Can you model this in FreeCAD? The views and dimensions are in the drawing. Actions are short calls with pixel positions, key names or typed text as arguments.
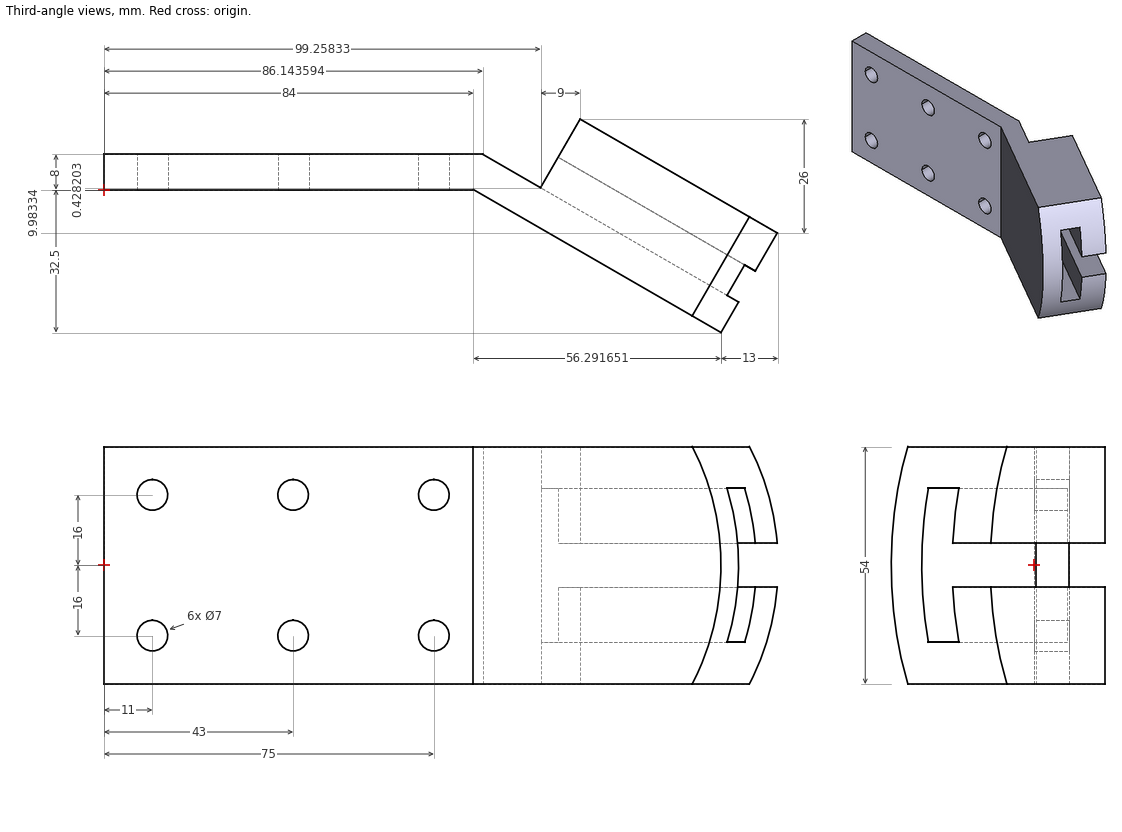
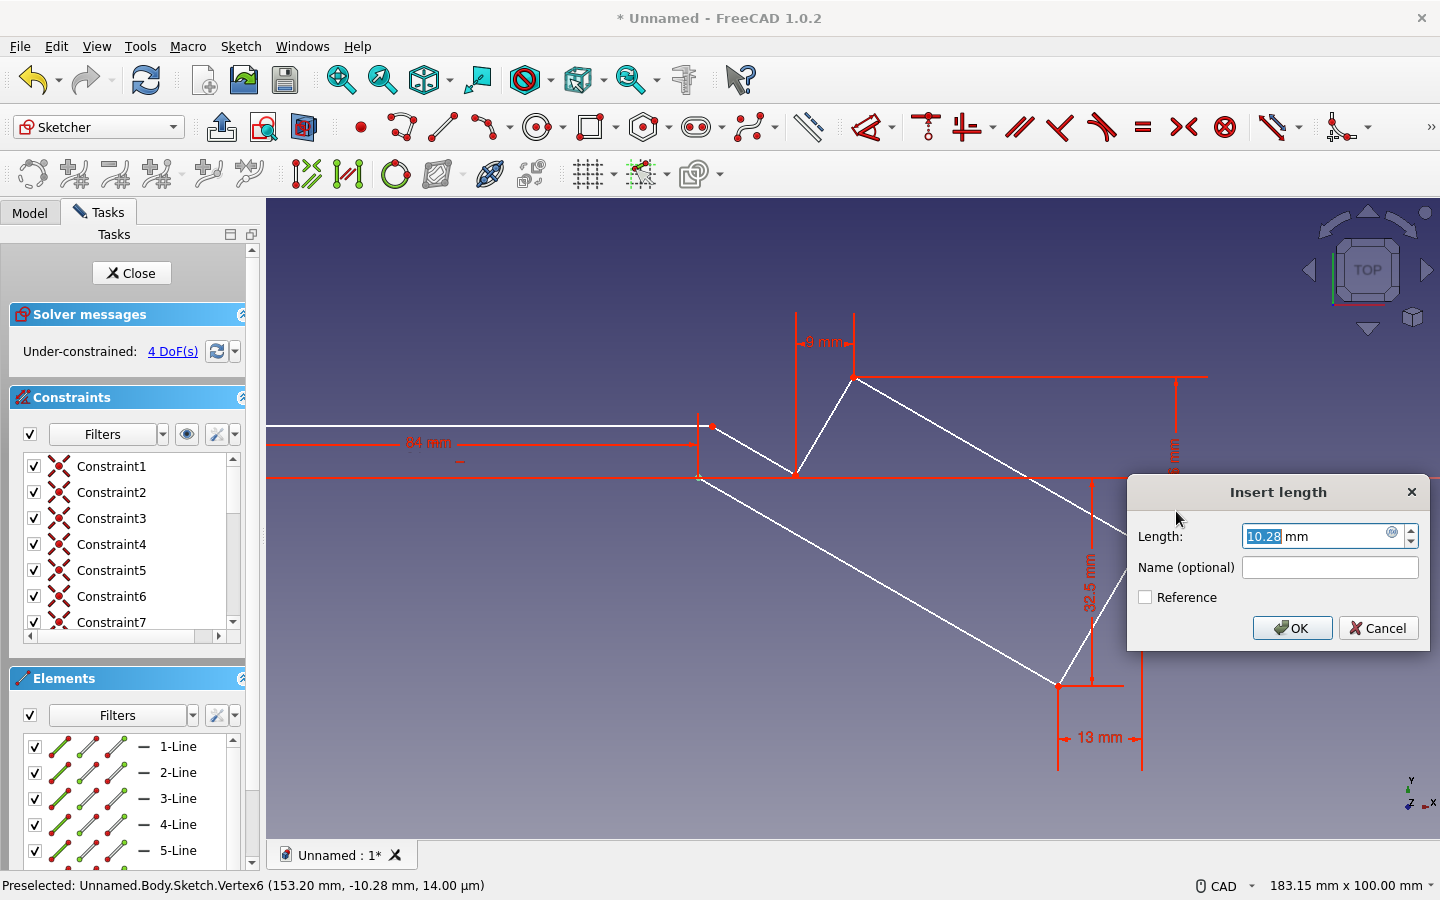
text(9.98334)
key(Return)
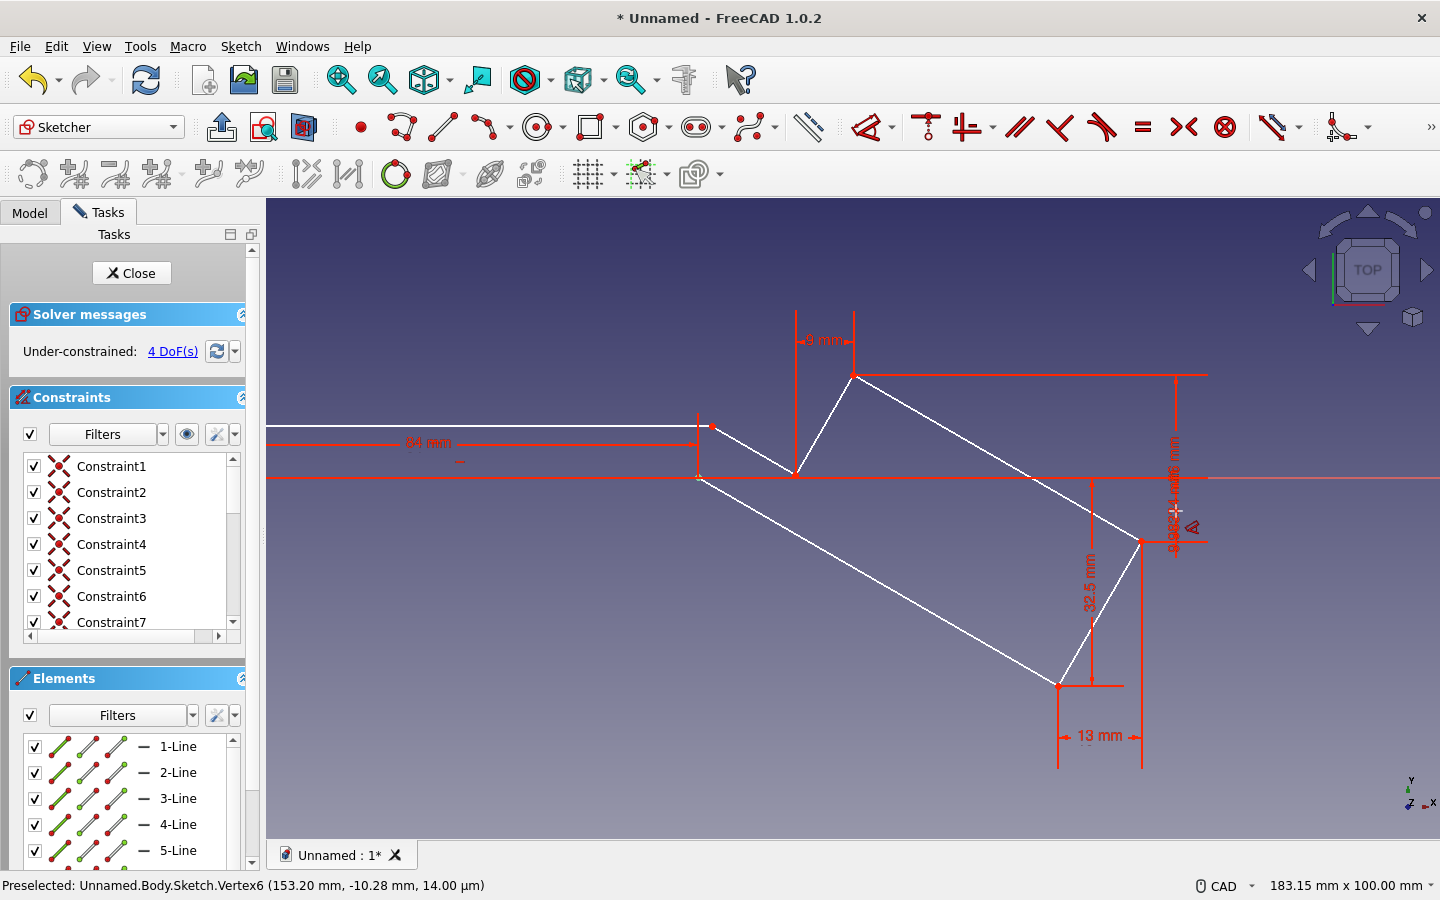
click(546, 426)
click(503, 392)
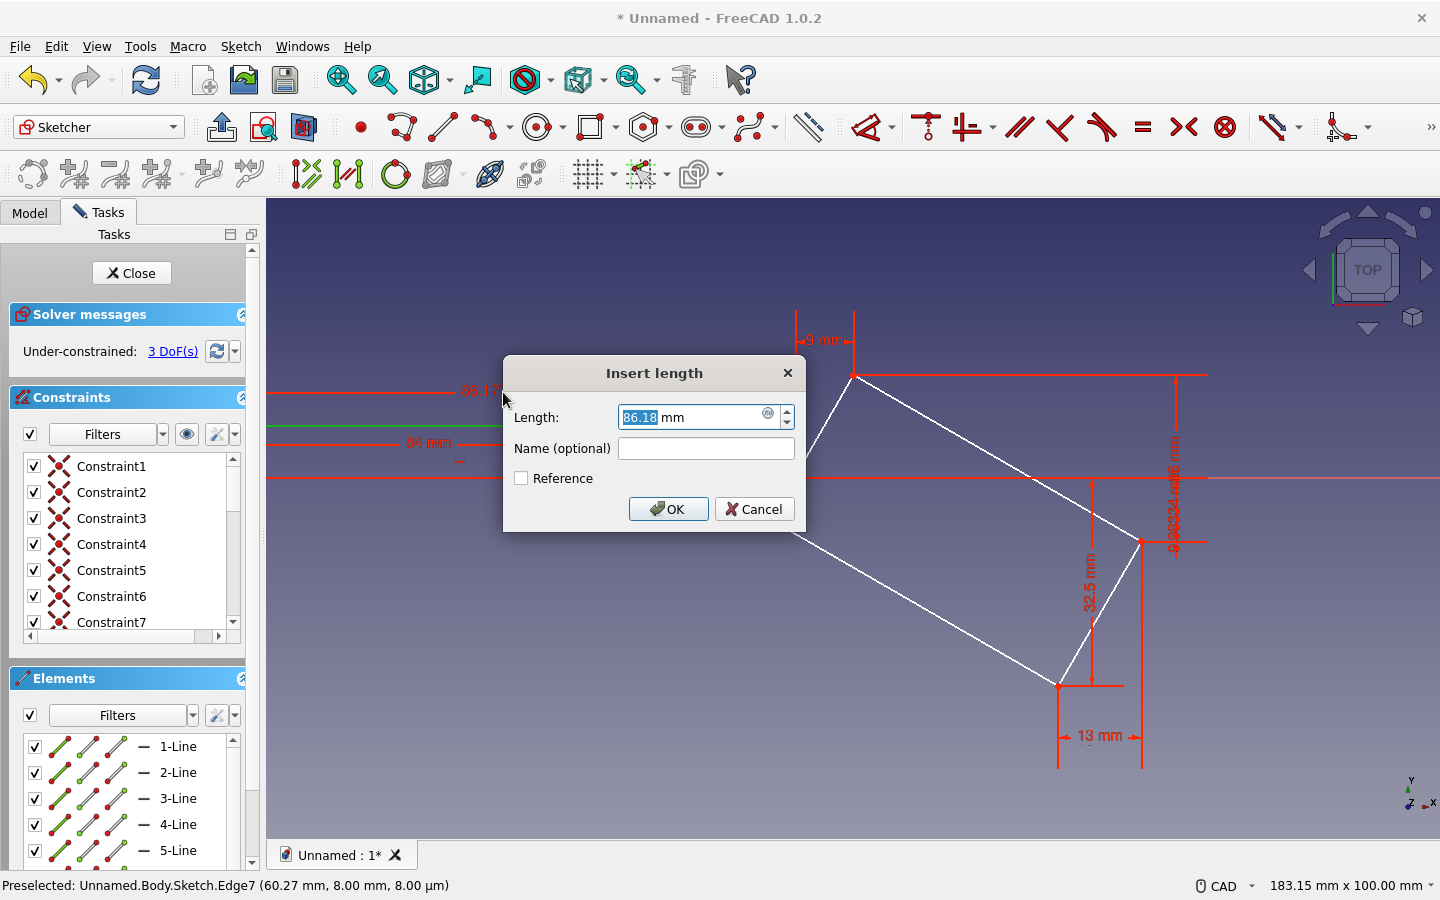
text(86.143594)
key(Return)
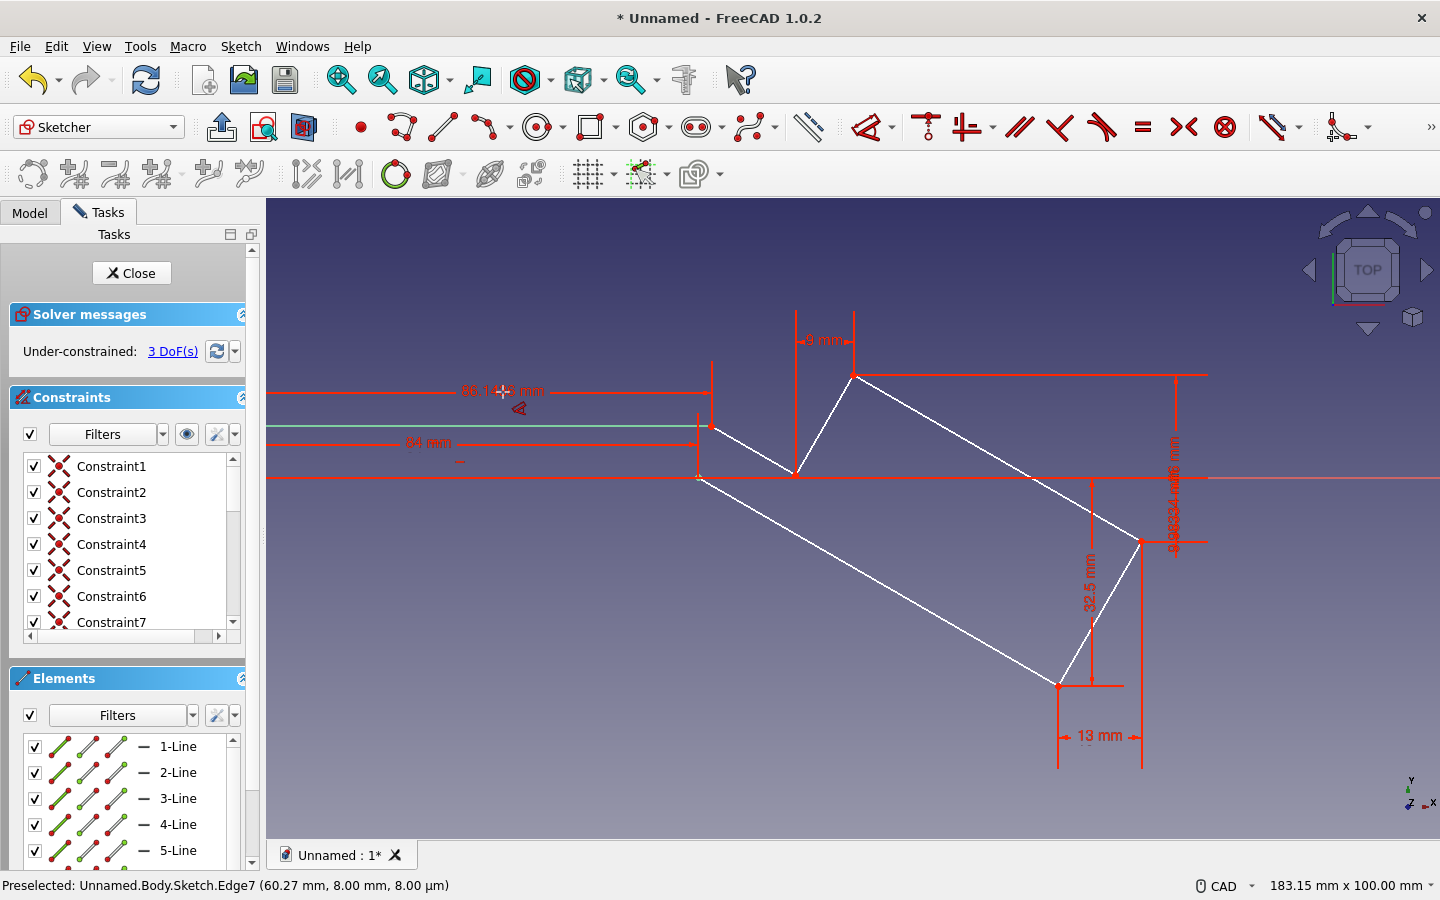
click(796, 475)
click(545, 441)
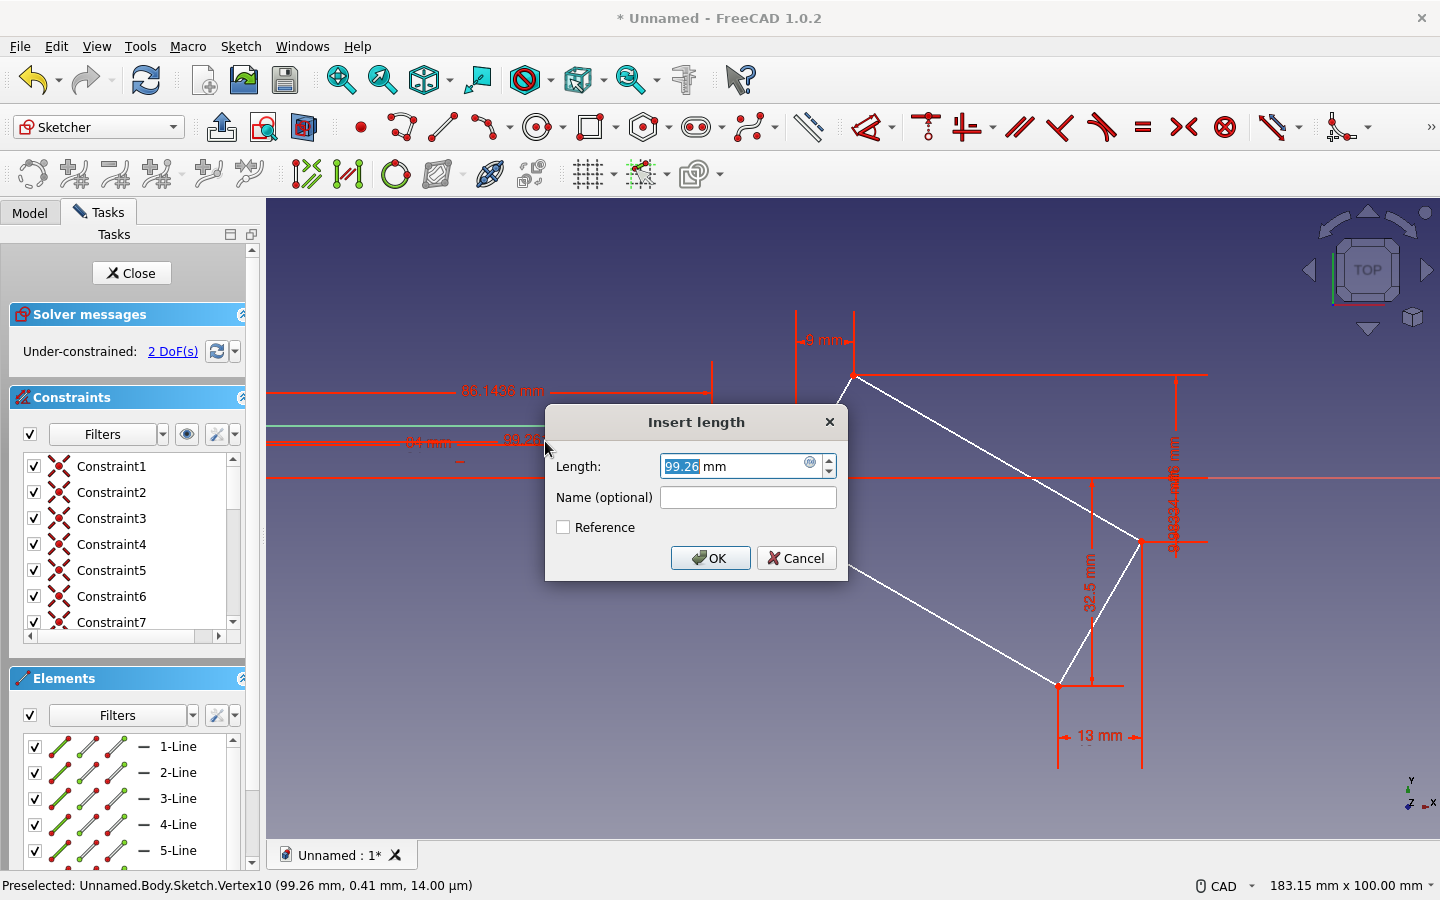
text(99.25833)
key(Return)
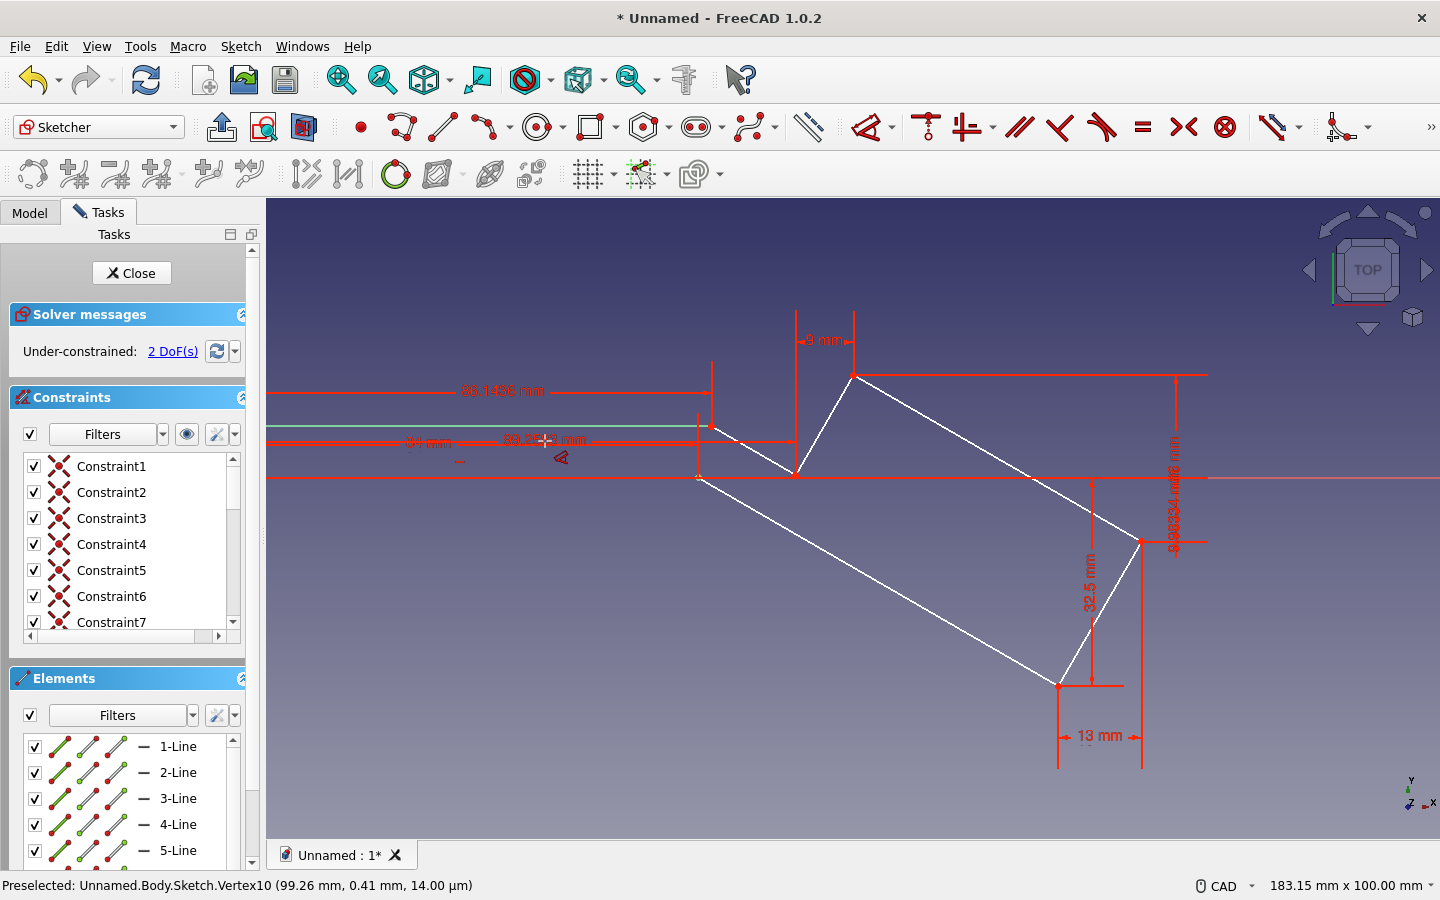
scroll(796, 475, up, 14)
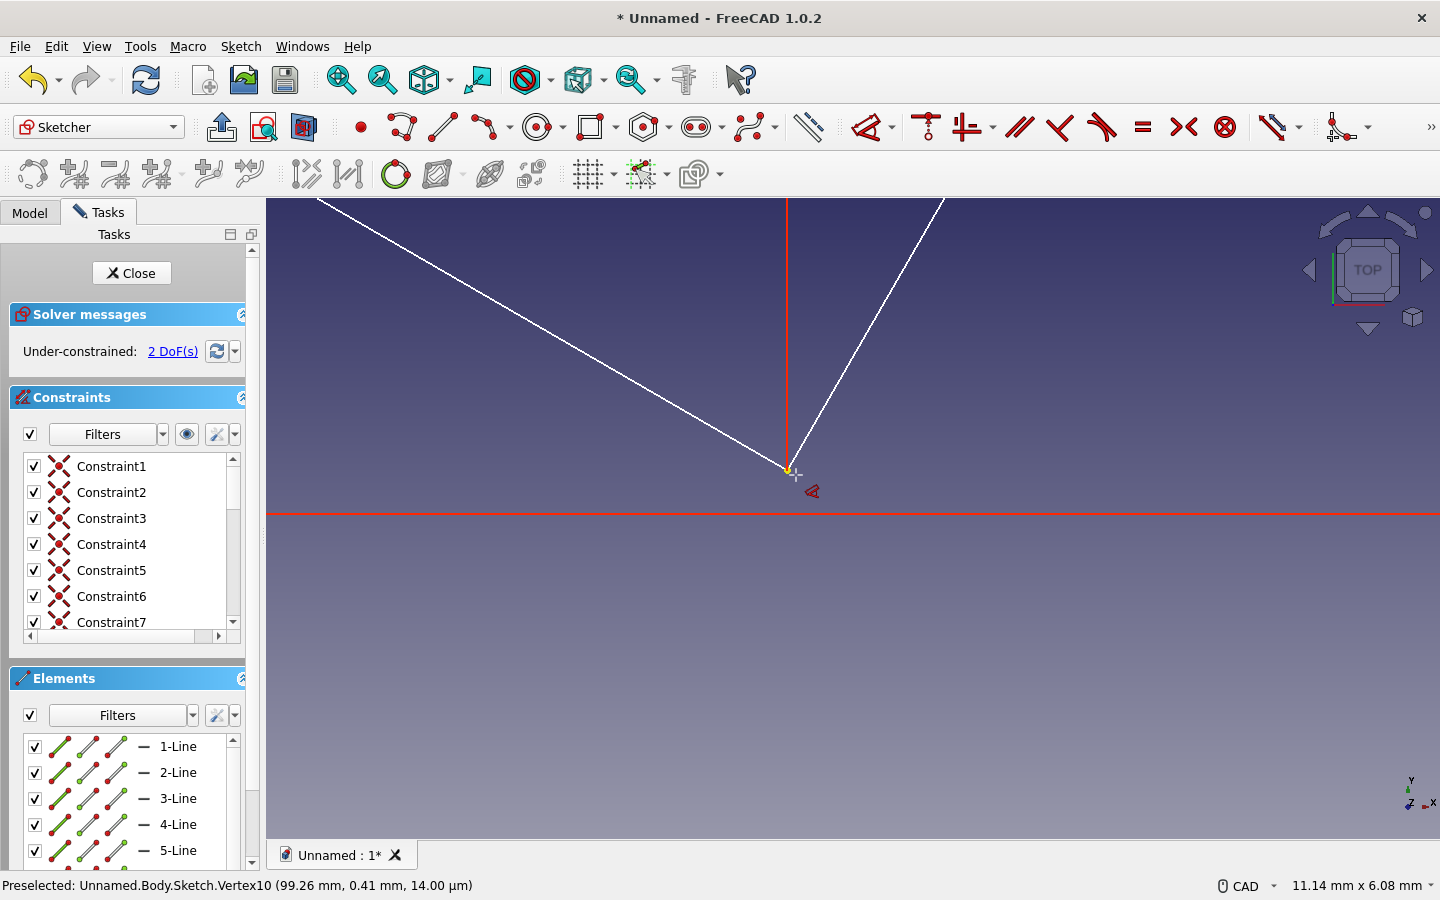
click(787, 471)
click(821, 492)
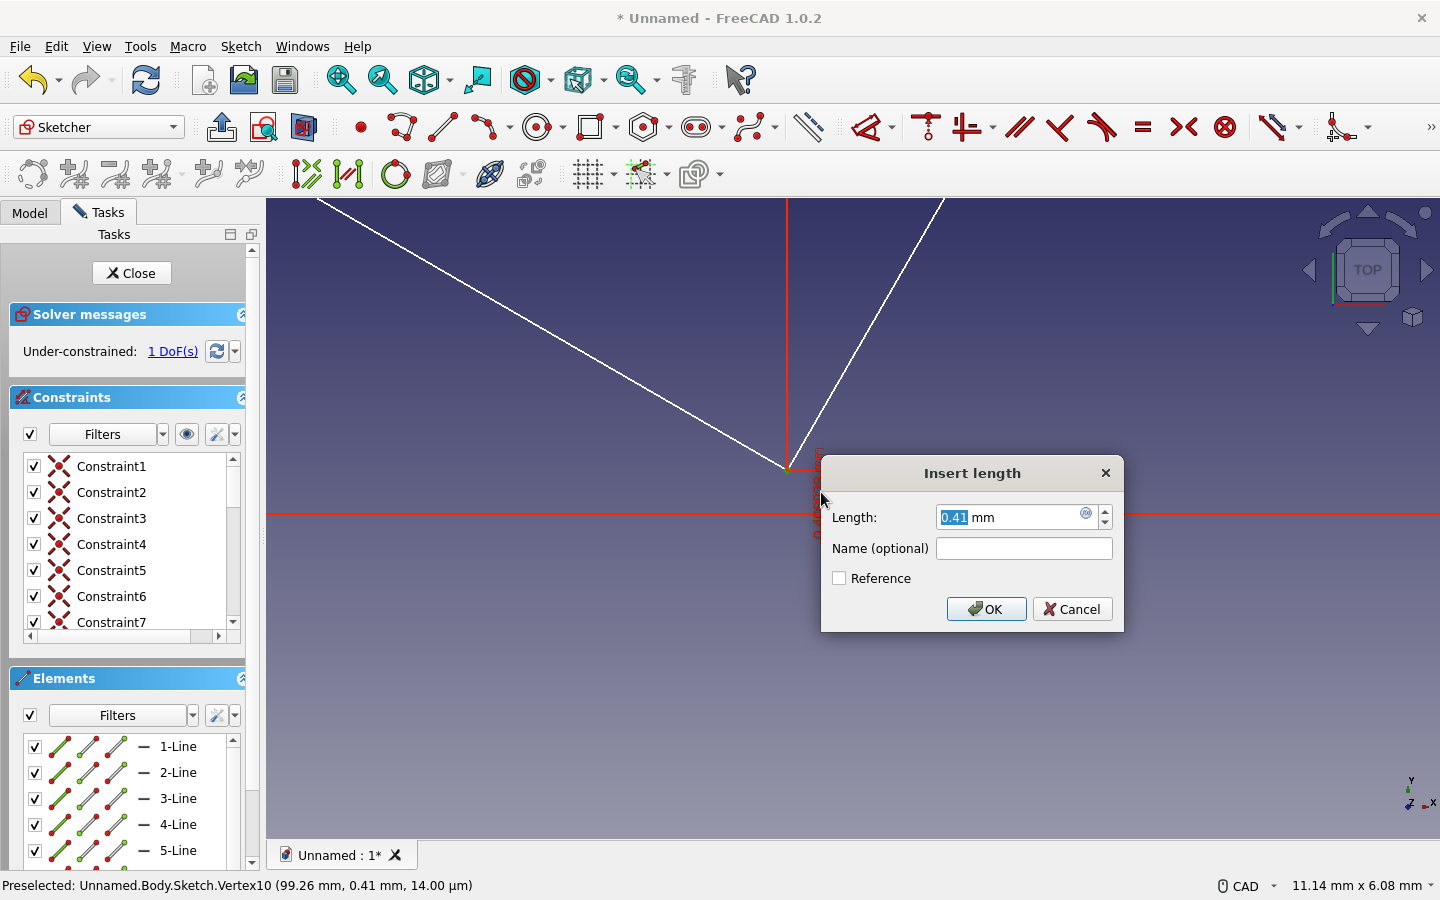
text(0.428203)
key(Return)